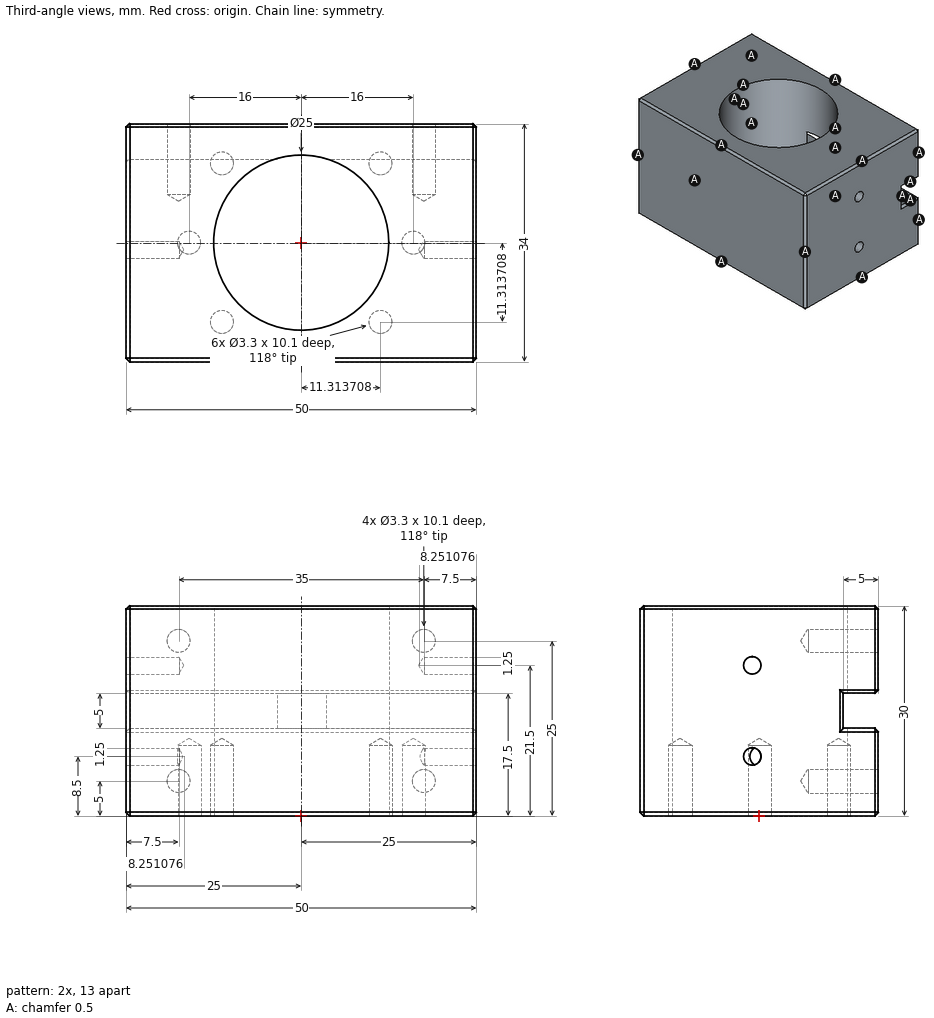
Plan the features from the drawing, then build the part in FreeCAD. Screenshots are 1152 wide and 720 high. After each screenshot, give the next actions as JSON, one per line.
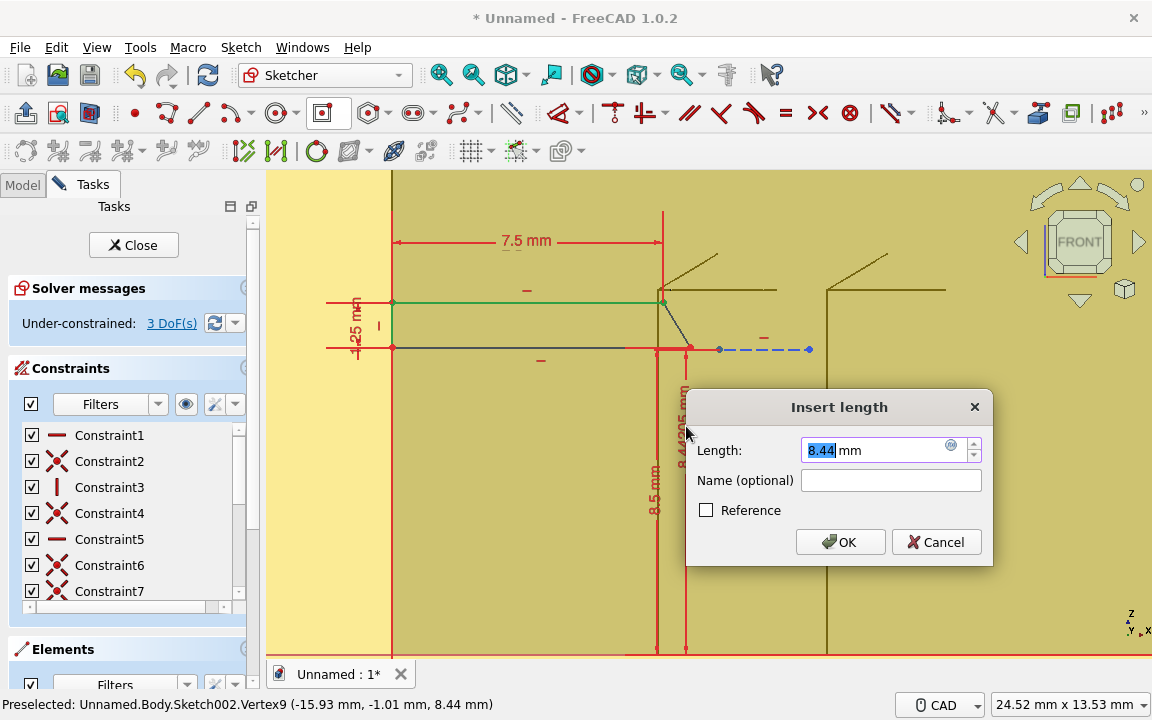
{"action": "type", "text": "8.5"}
{"action": "key", "text": "Return"}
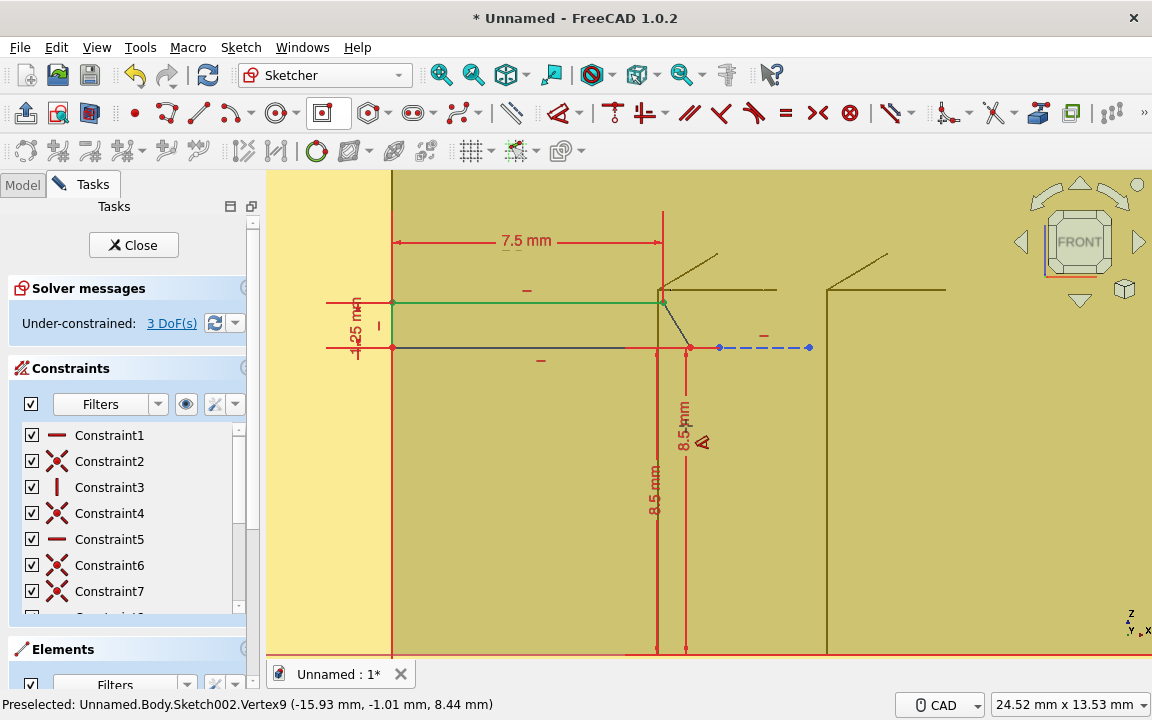
{"action": "left_click", "coordinate": [601, 348]}
{"action": "left_click", "coordinate": [541, 382]}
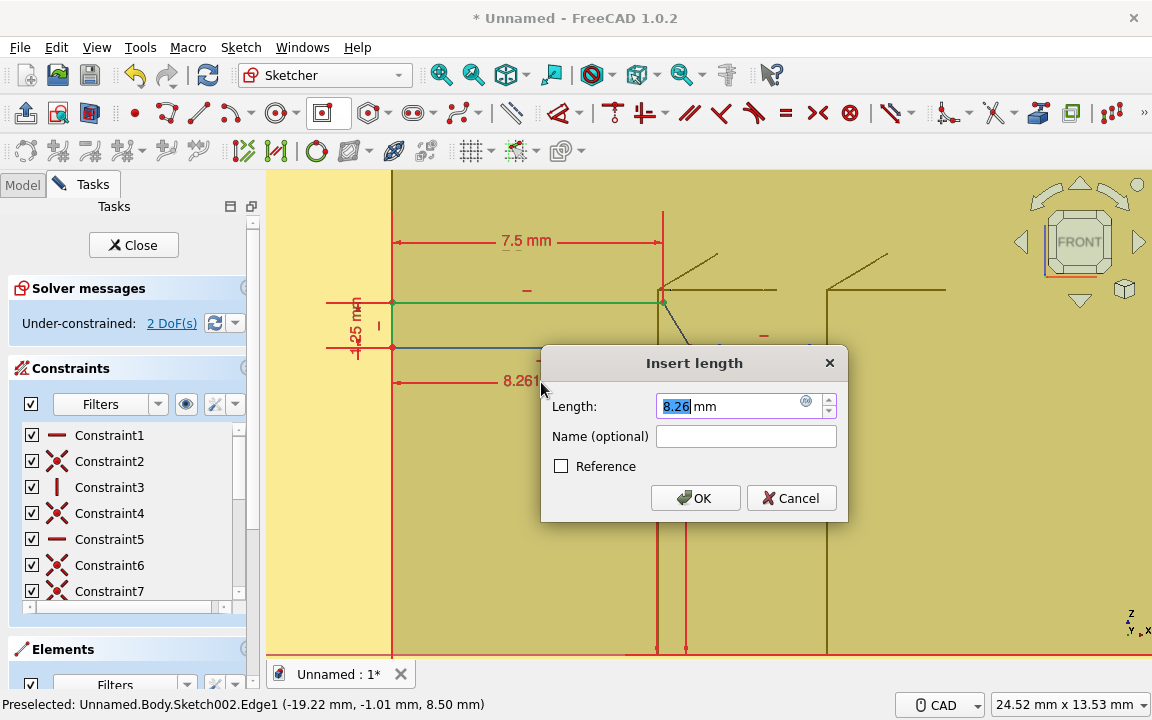
{"action": "type", "text": "8.251076"}
{"action": "key", "text": "Return"}
{"action": "key", "text": "Escape"}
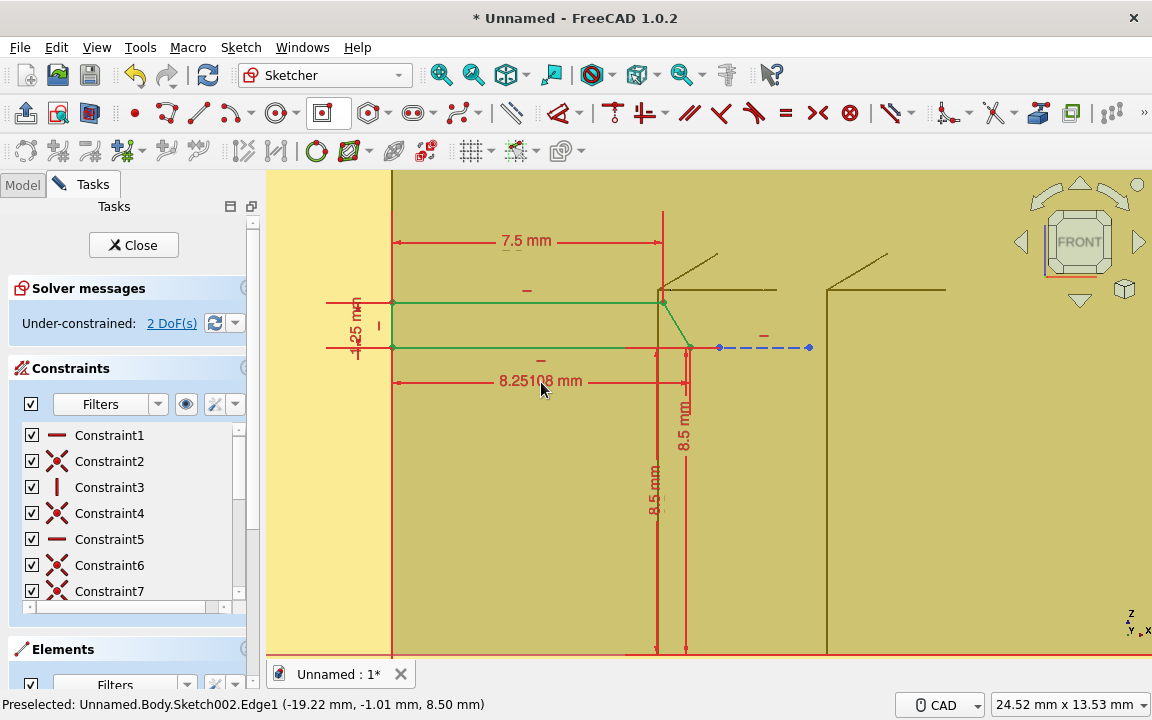
{"action": "left_click", "coordinate": [134, 245]}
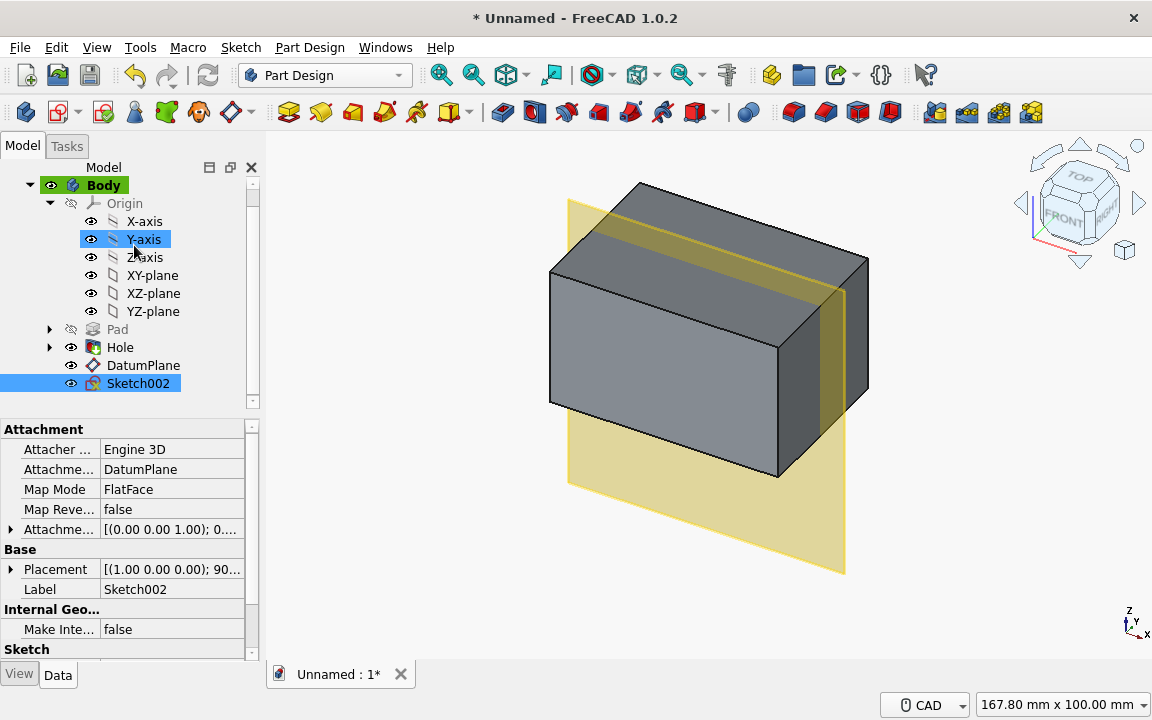
{"action": "left_click", "coordinate": [568, 112]}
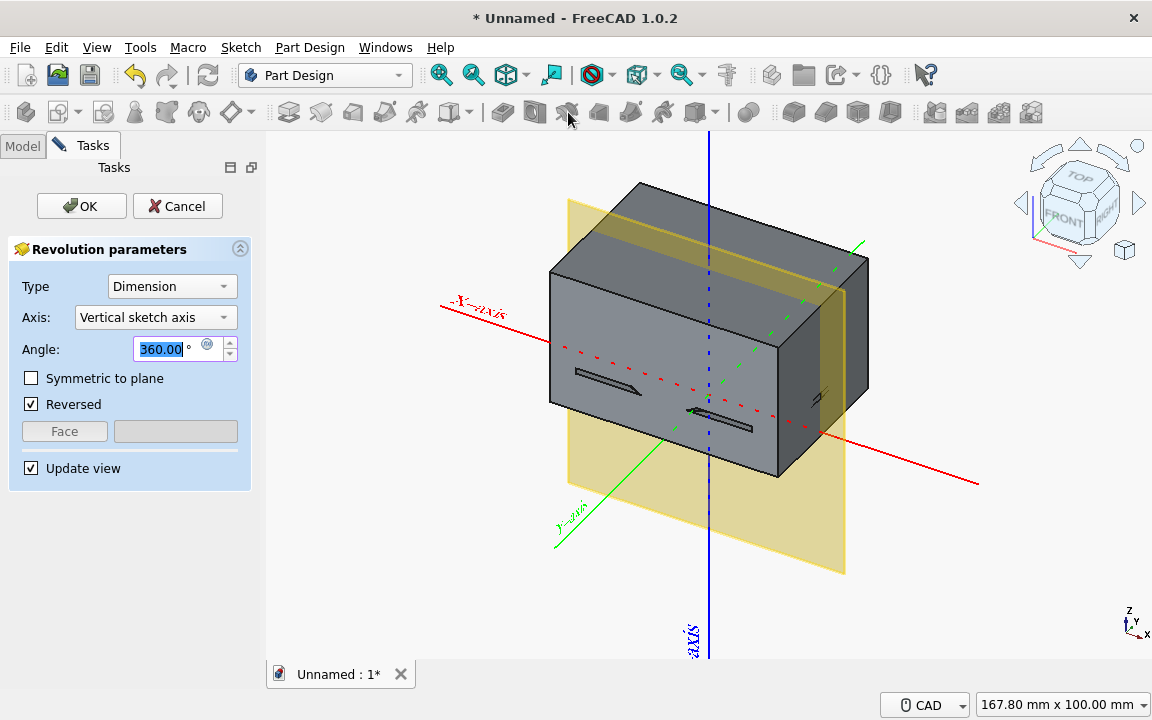
{"action": "left_click", "coordinate": [156, 318]}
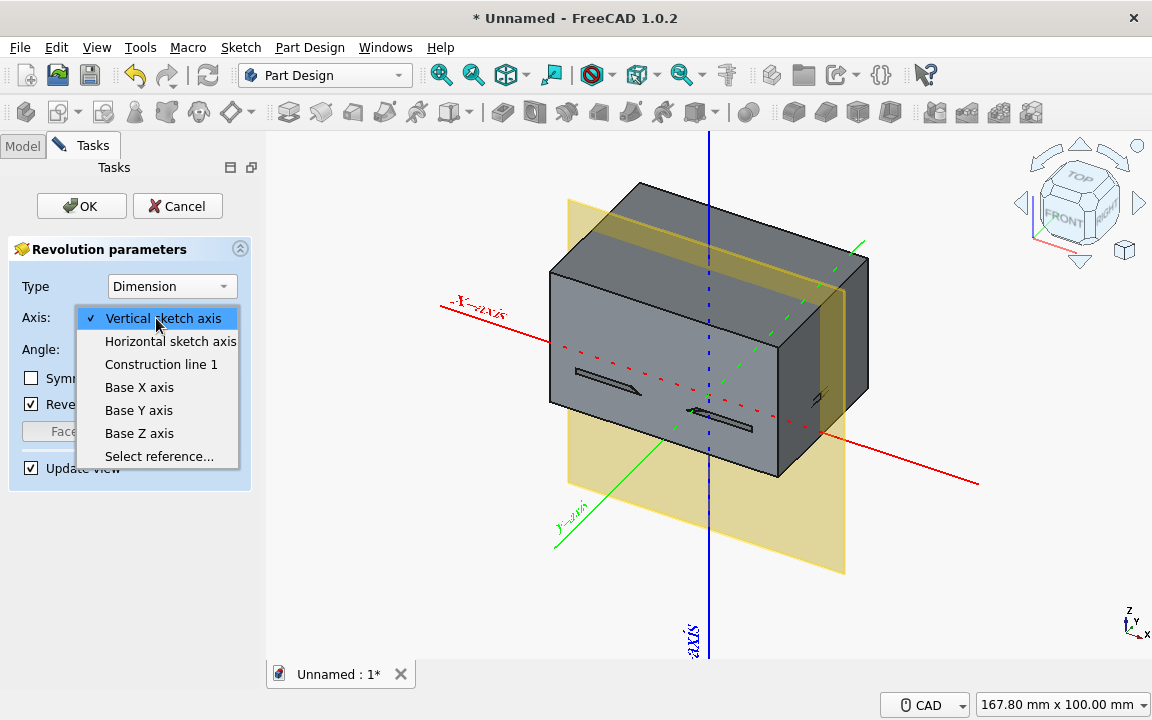
{"action": "left_click", "coordinate": [156, 364]}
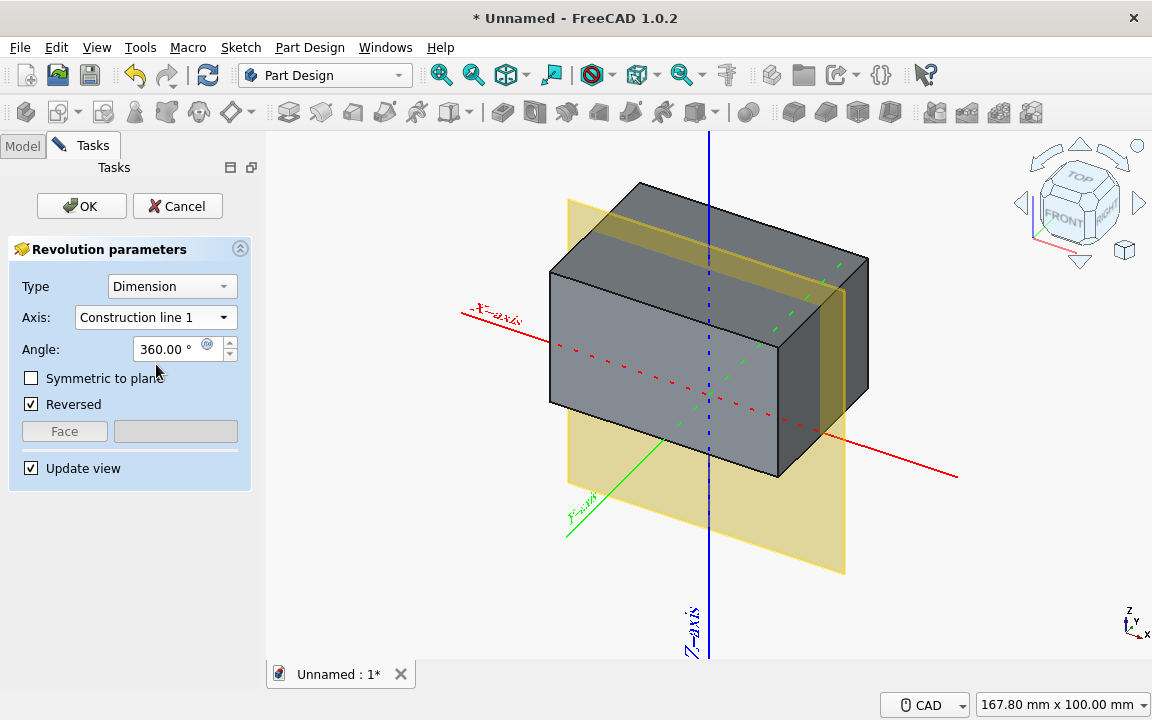
{"action": "left_click", "coordinate": [82, 206]}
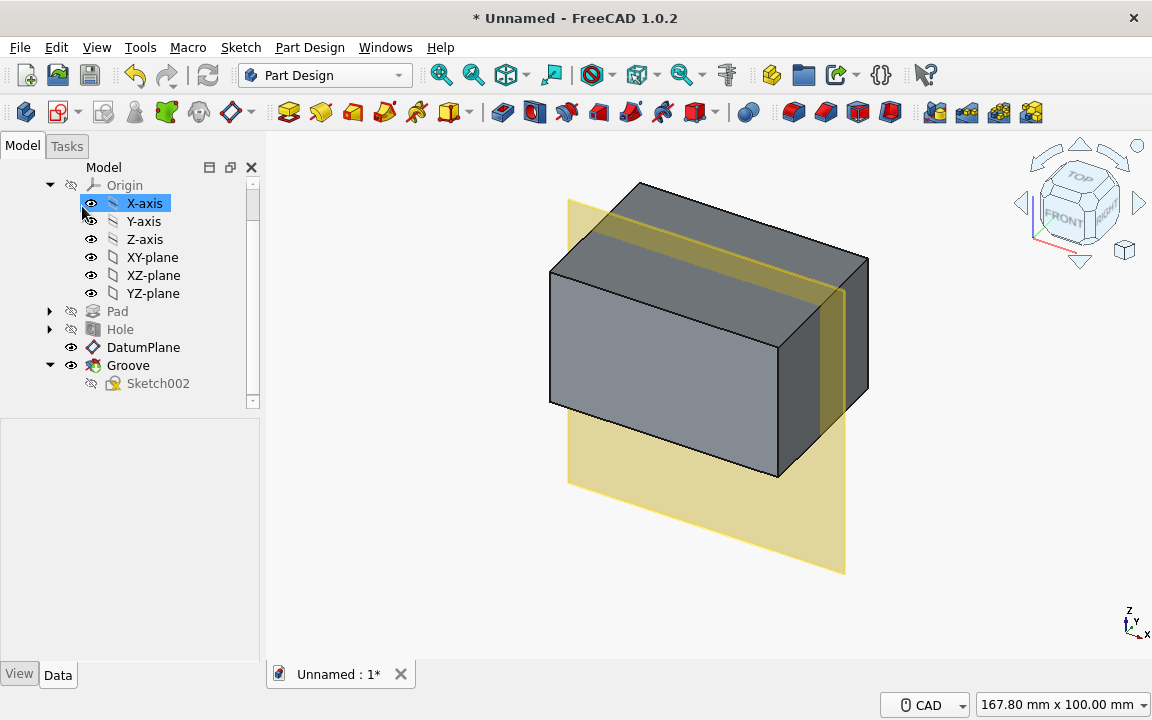
{"action": "left_click", "coordinate": [116, 347]}
{"action": "key", "text": "space"}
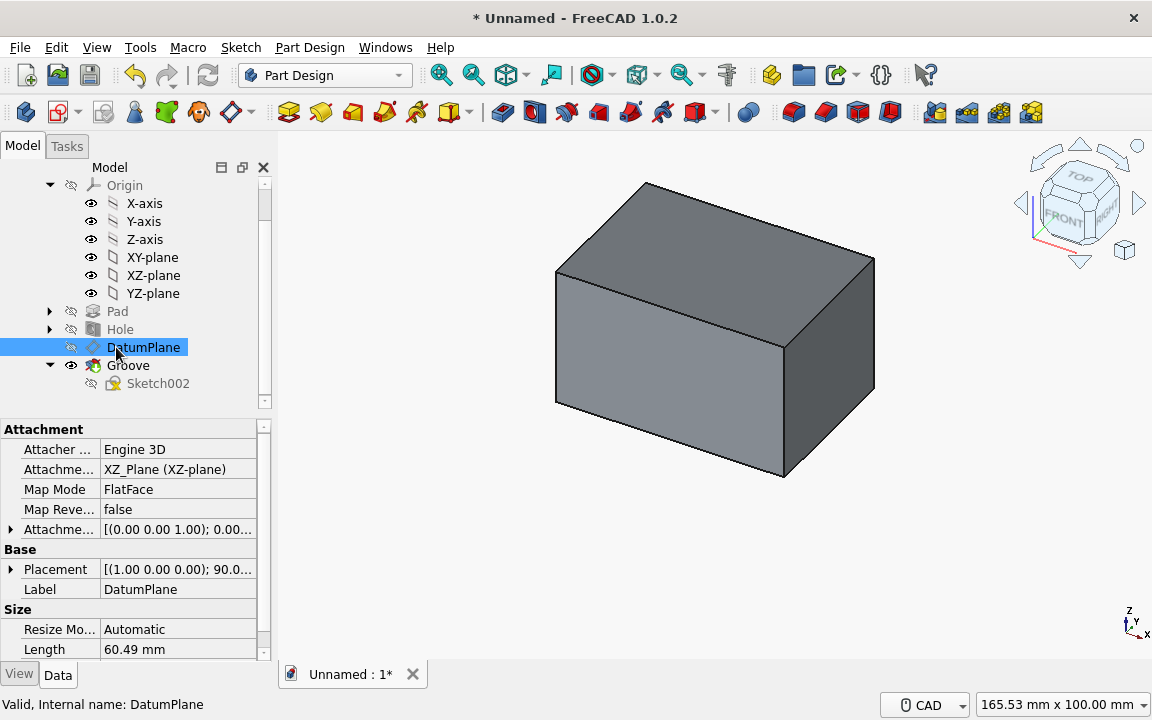
{"action": "left_click", "coordinate": [116, 365]}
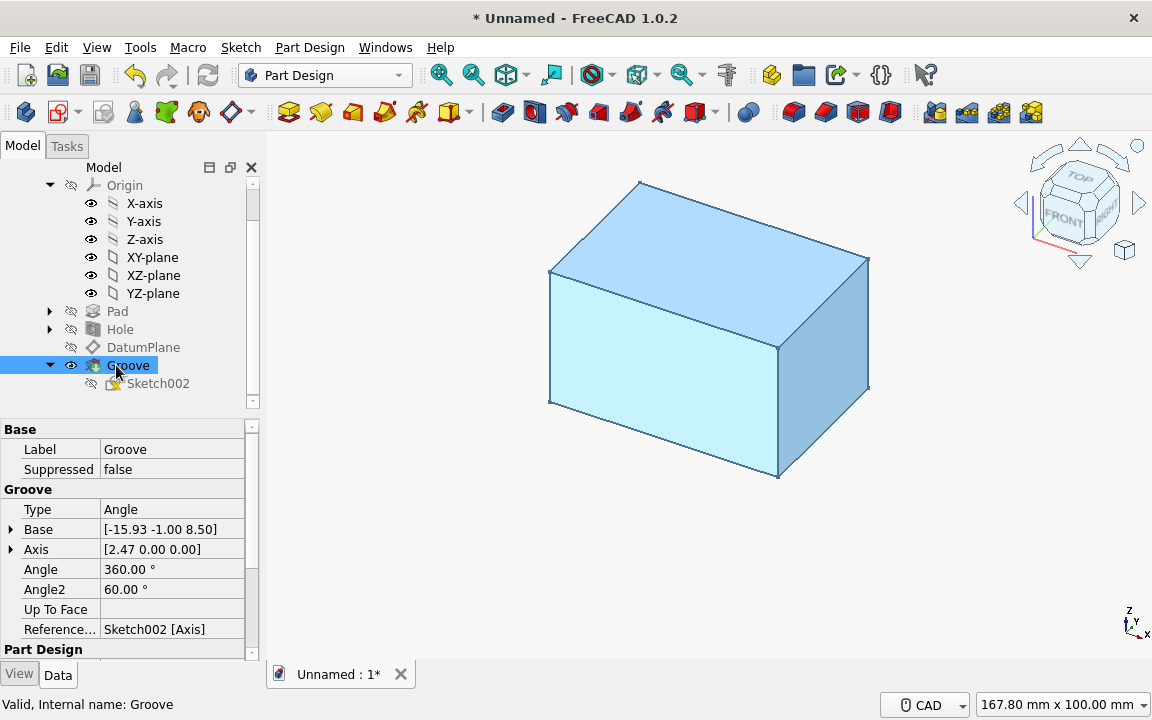
{"action": "left_click", "coordinate": [968, 112]}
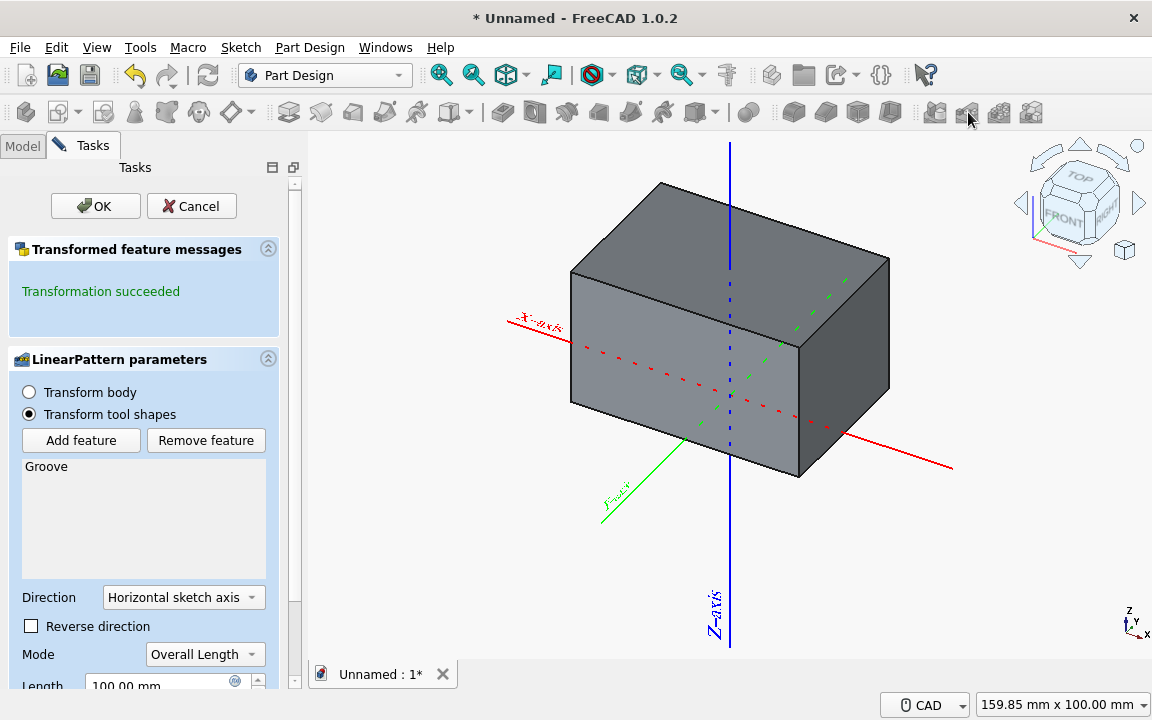
{"action": "left_click", "coordinate": [184, 598]}